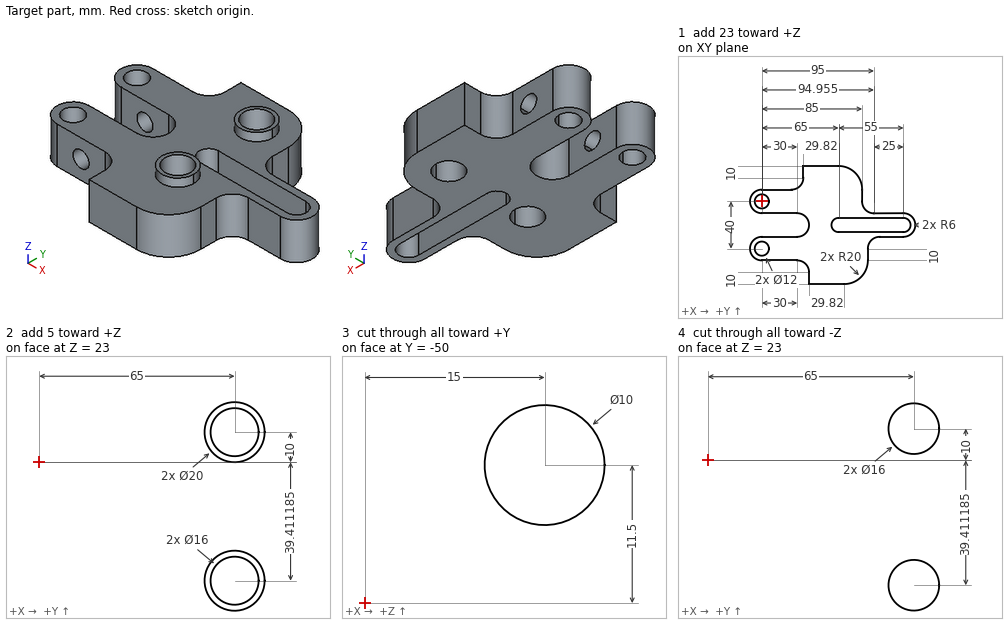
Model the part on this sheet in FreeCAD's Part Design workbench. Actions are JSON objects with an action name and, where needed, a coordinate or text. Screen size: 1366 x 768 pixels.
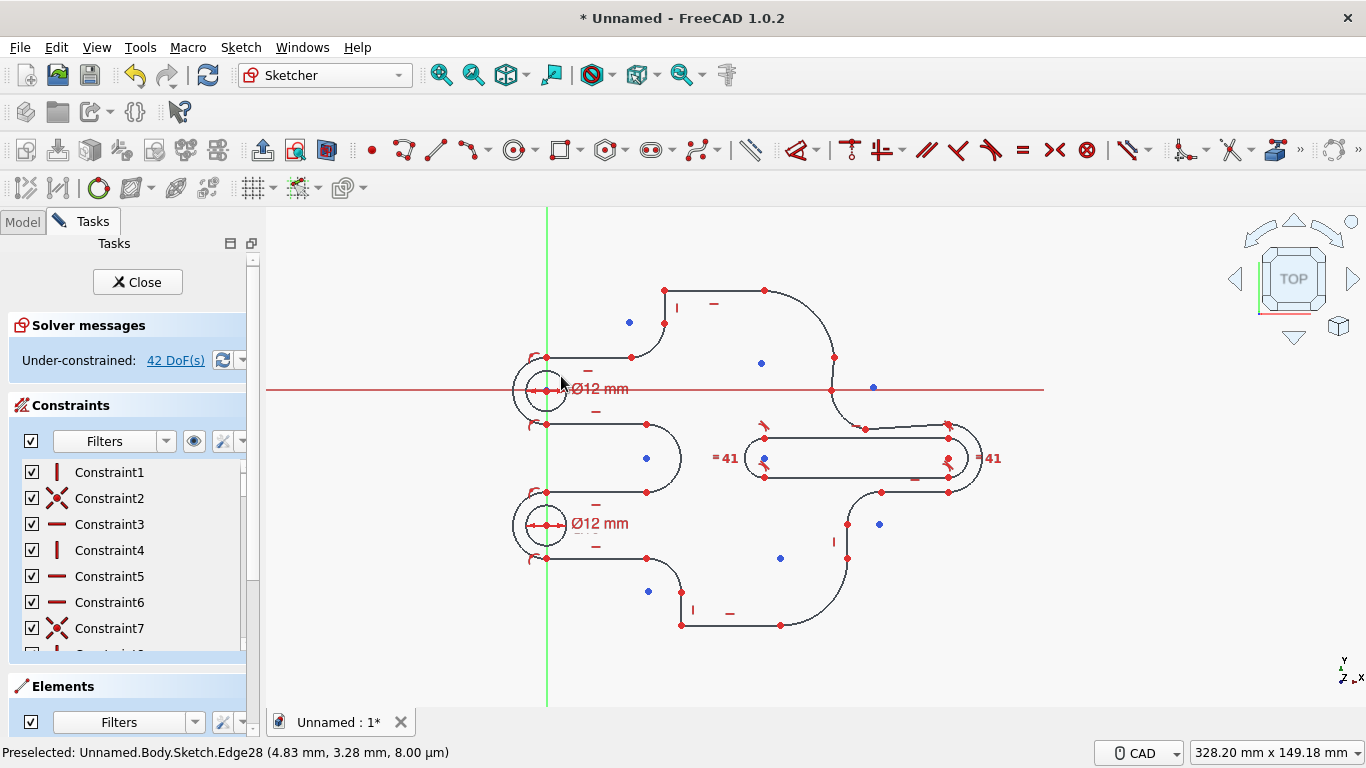
{"action": "scroll", "coordinate": [681, 603], "scroll_direction": "up", "scroll_amount": 2}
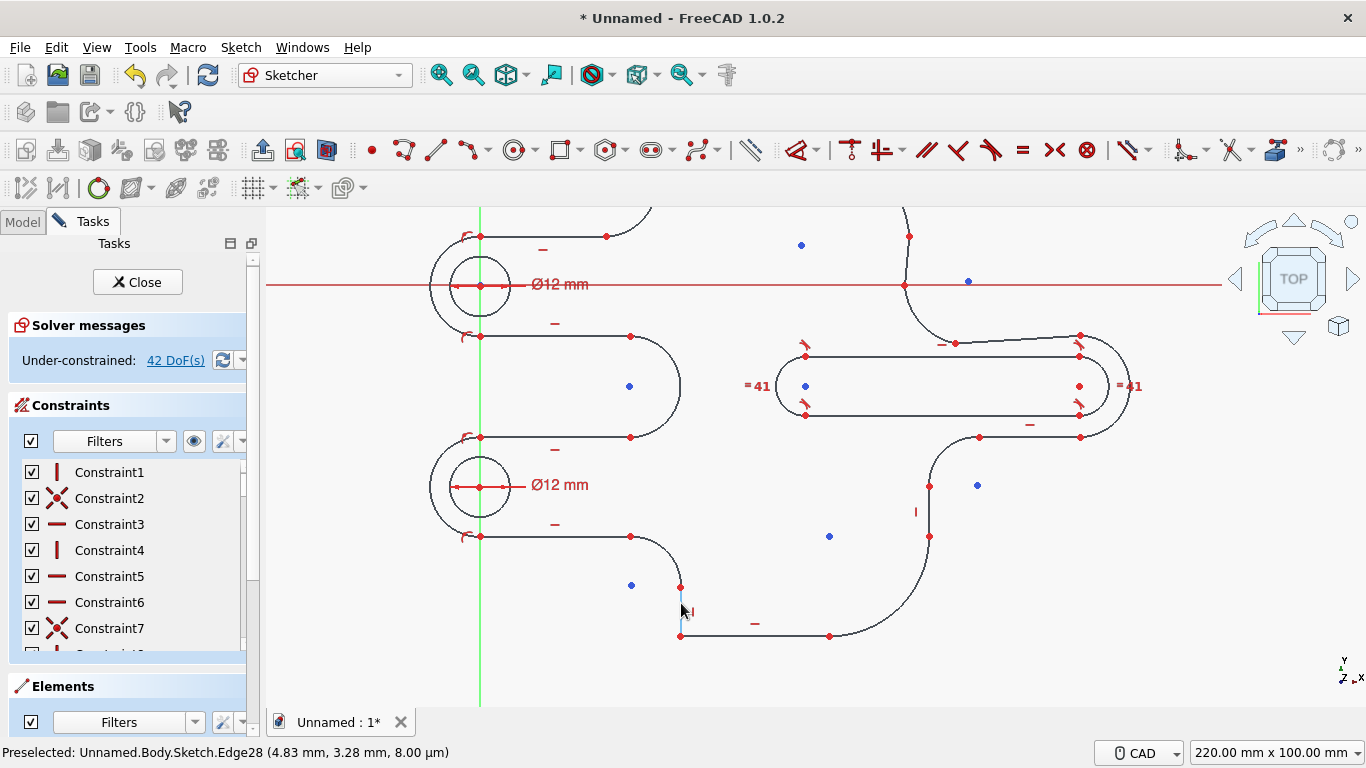
{"action": "left_click", "coordinate": [681, 602]}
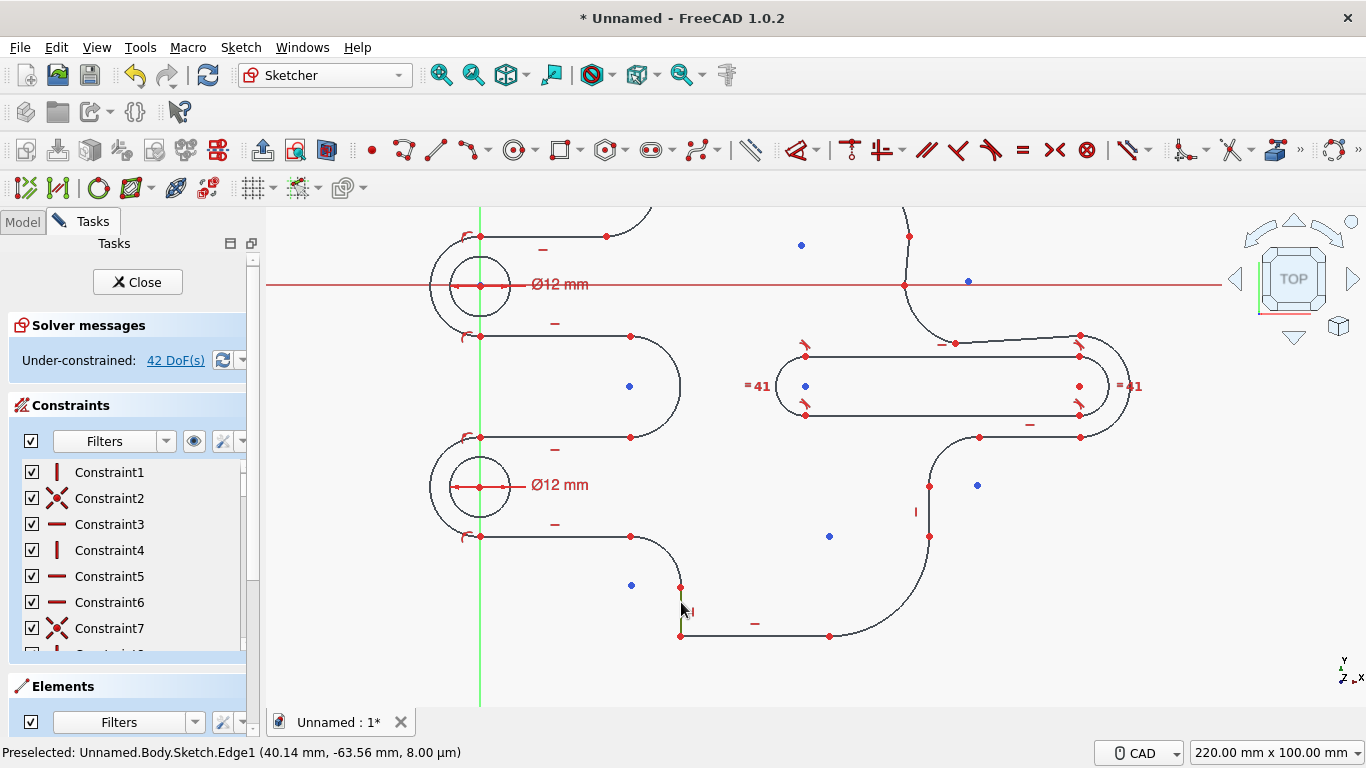
{"action": "left_click", "coordinate": [676, 564]}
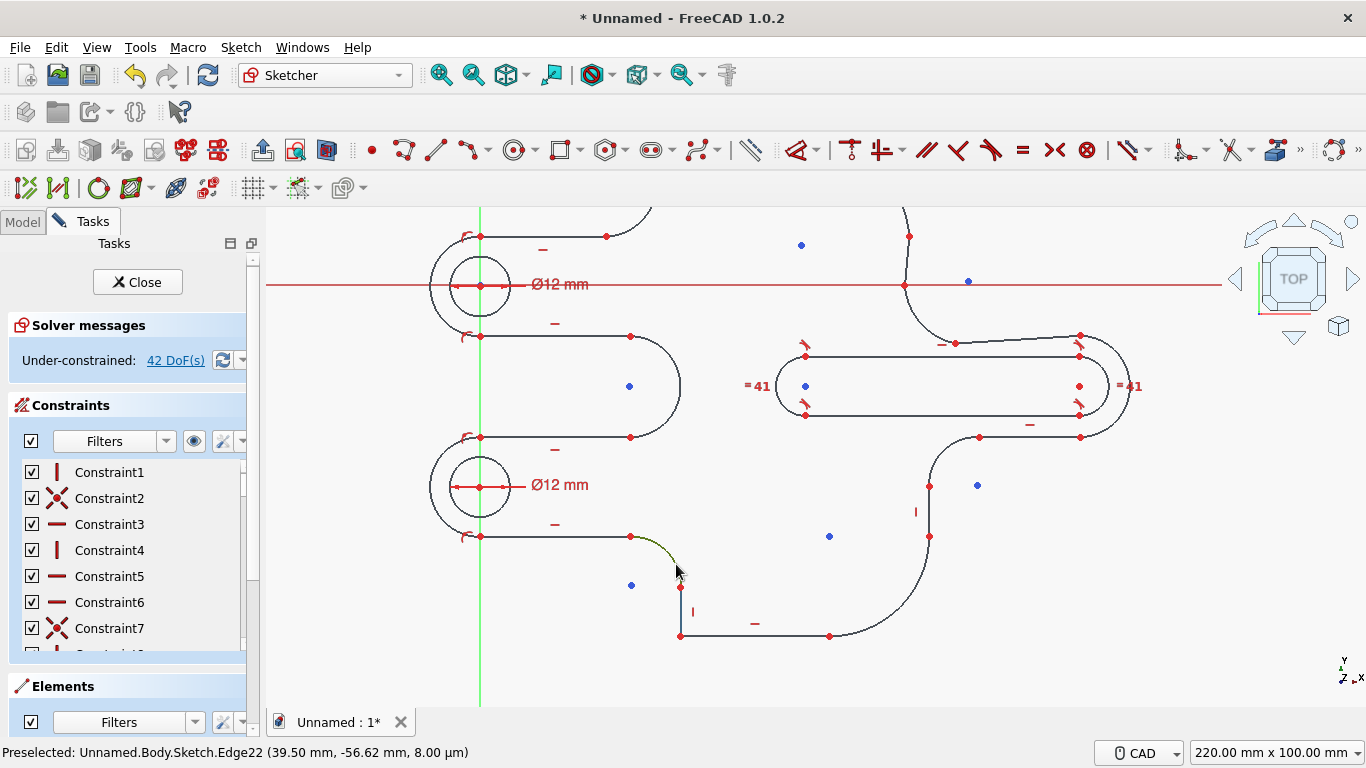
{"action": "left_click", "coordinate": [992, 150]}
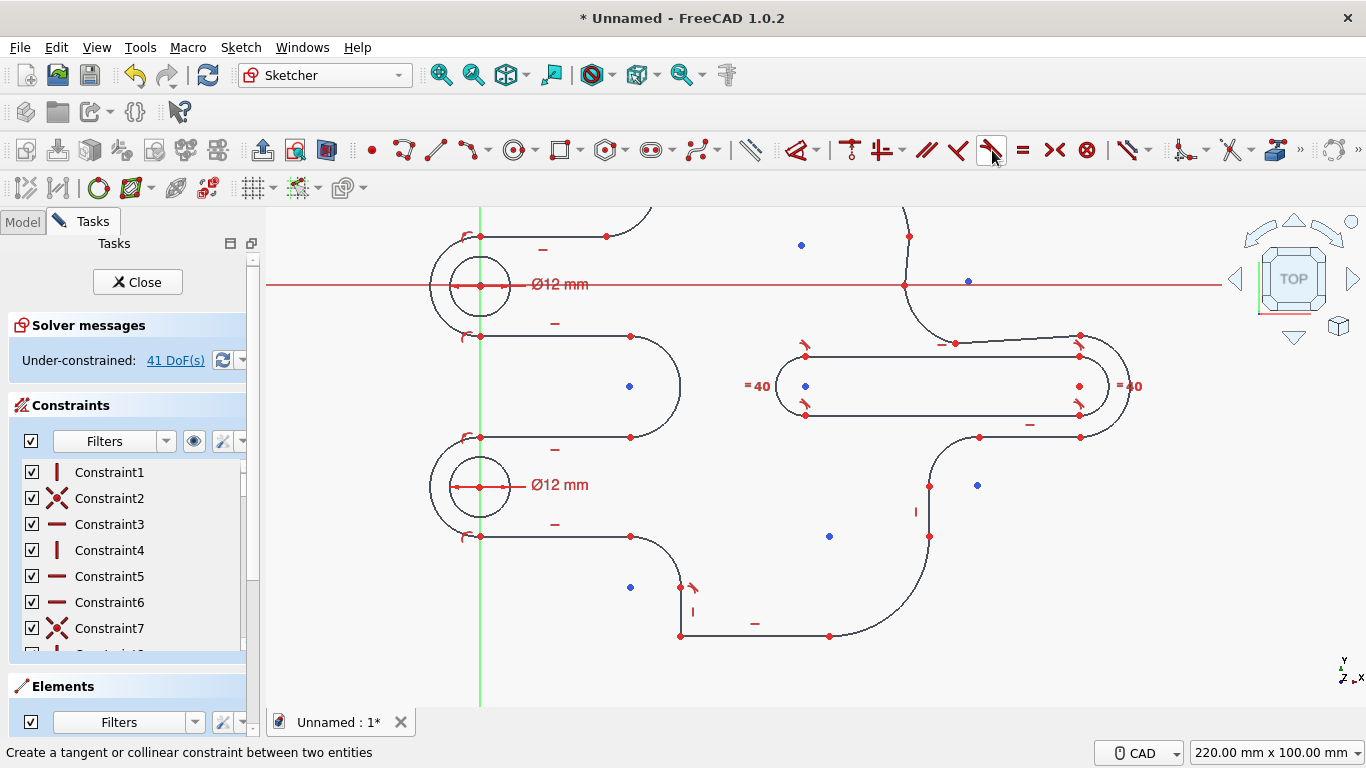
{"action": "left_click", "coordinate": [725, 636]}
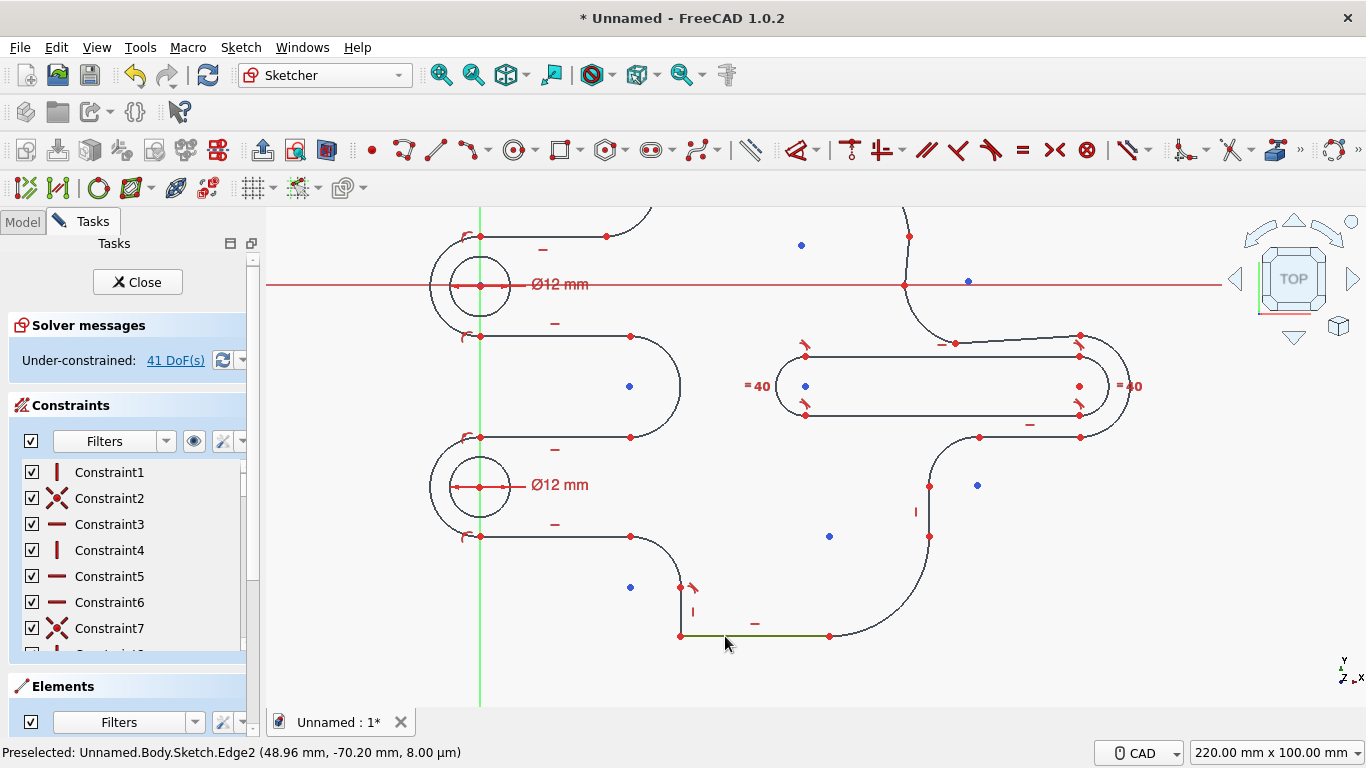
{"action": "left_click", "coordinate": [875, 625]}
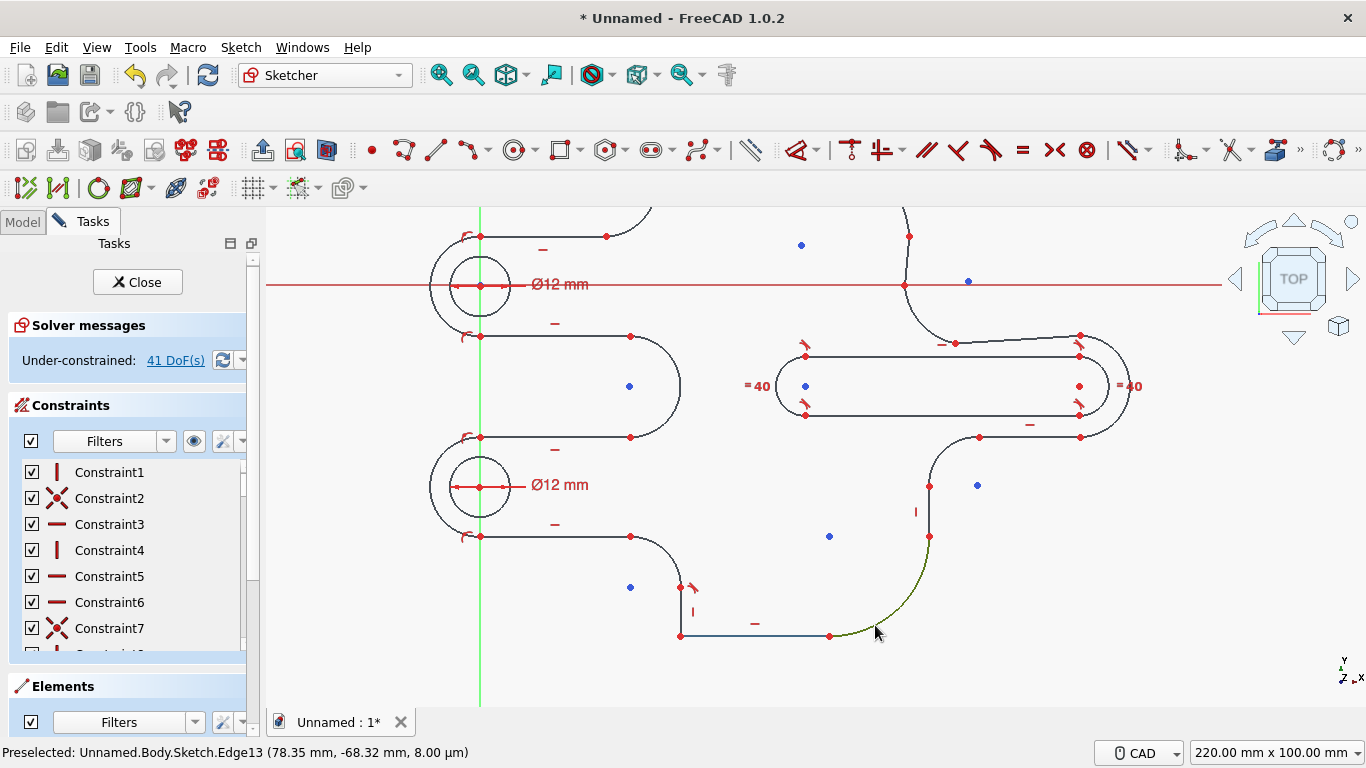
{"action": "key", "text": "t"}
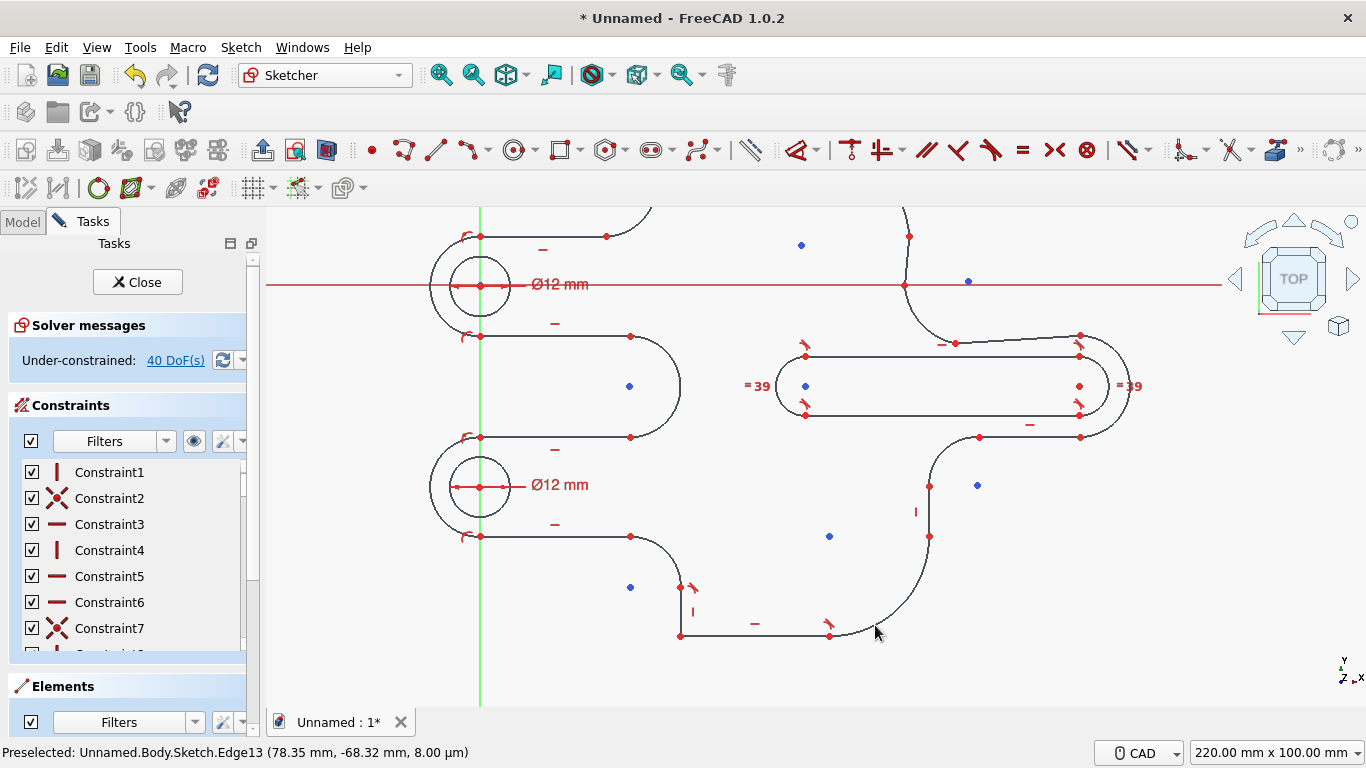
{"action": "left_click", "coordinate": [929, 522]}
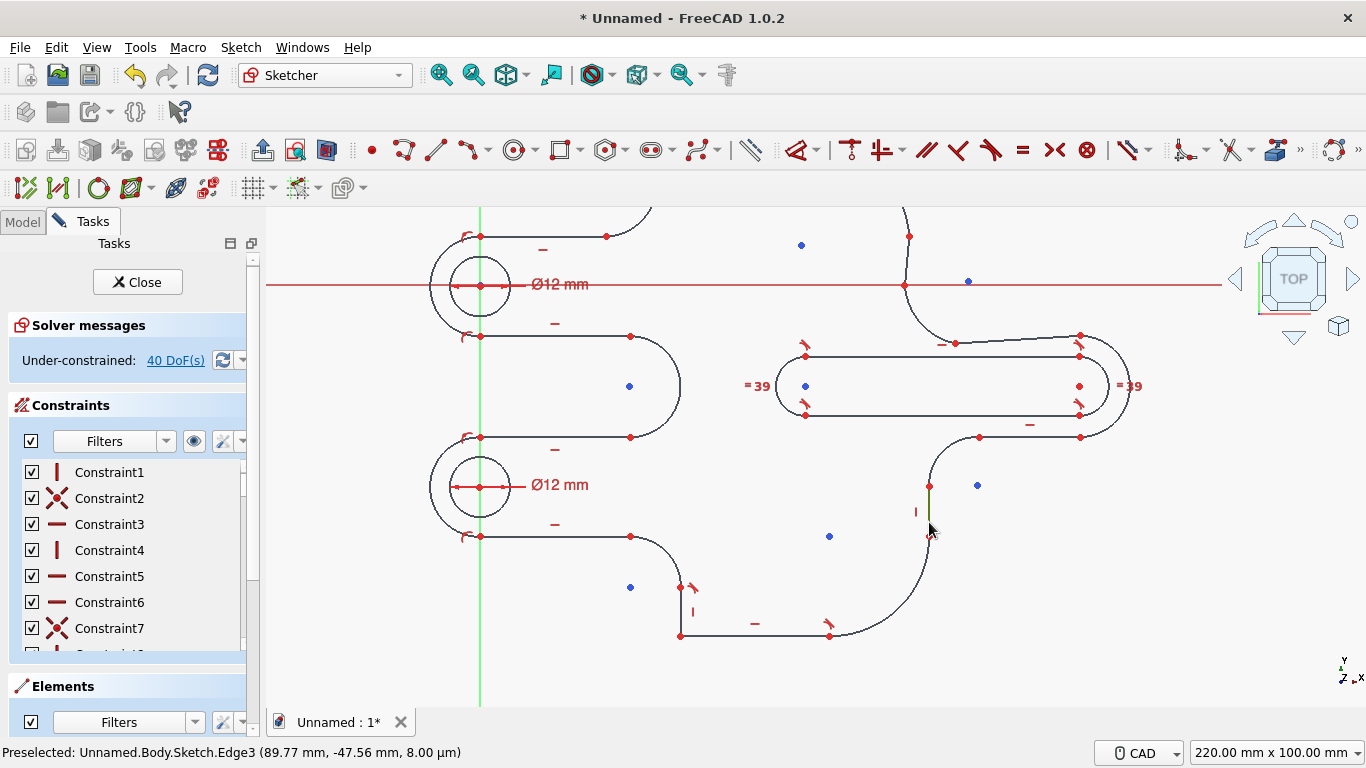
{"action": "left_click", "coordinate": [875, 625]}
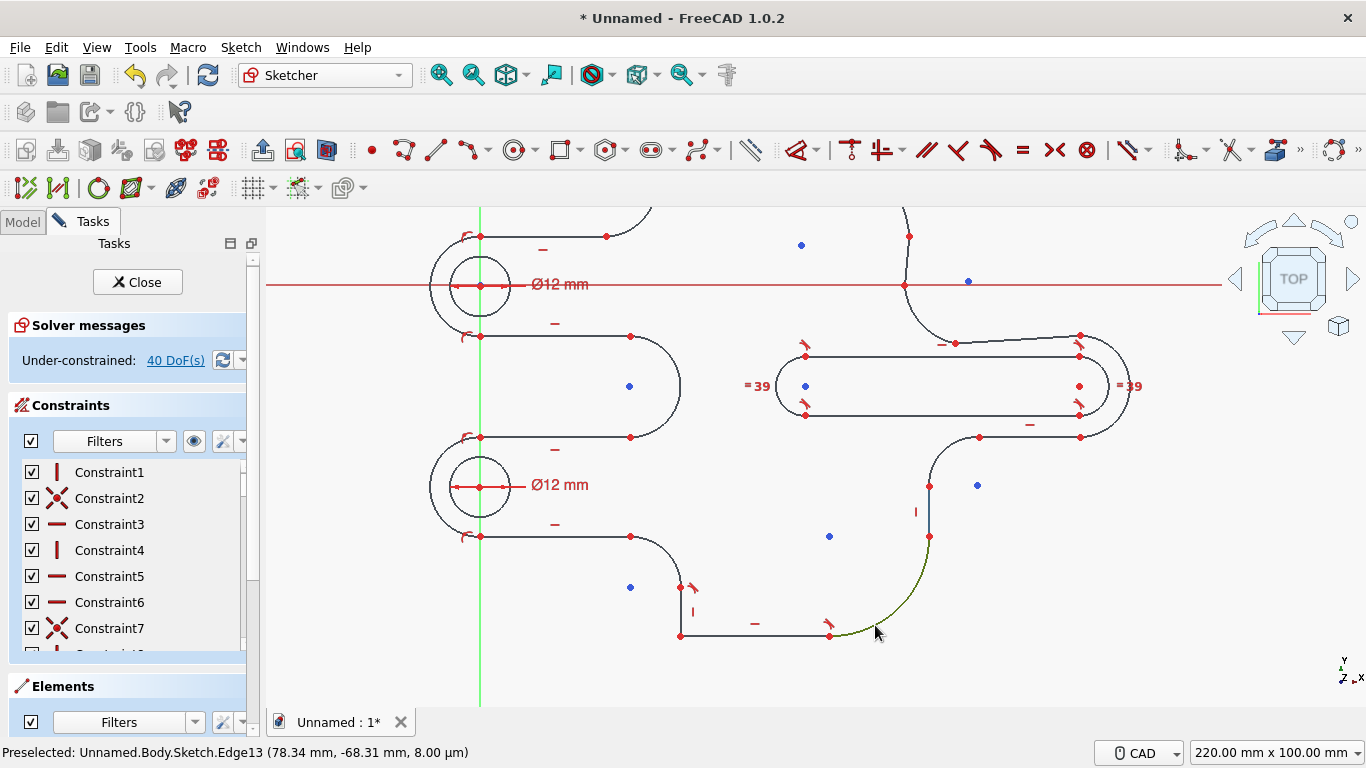
{"action": "left_click", "coordinate": [992, 150]}